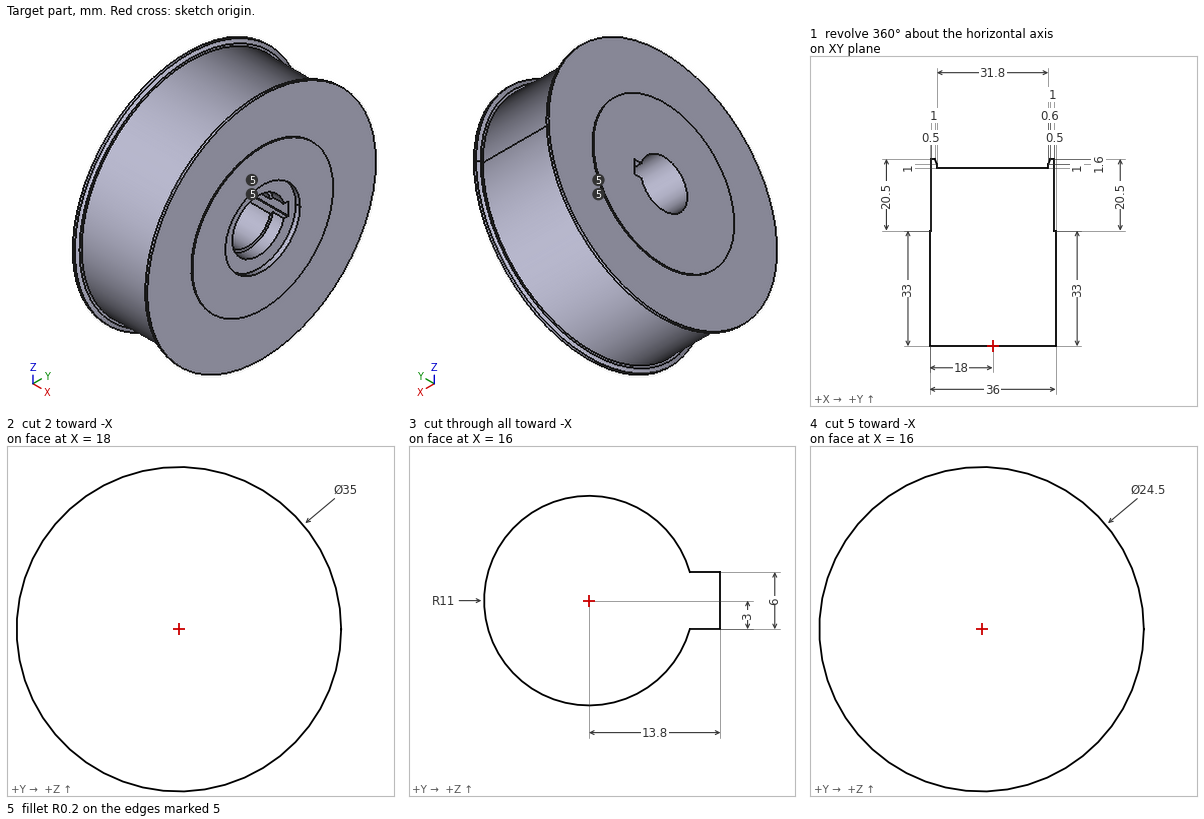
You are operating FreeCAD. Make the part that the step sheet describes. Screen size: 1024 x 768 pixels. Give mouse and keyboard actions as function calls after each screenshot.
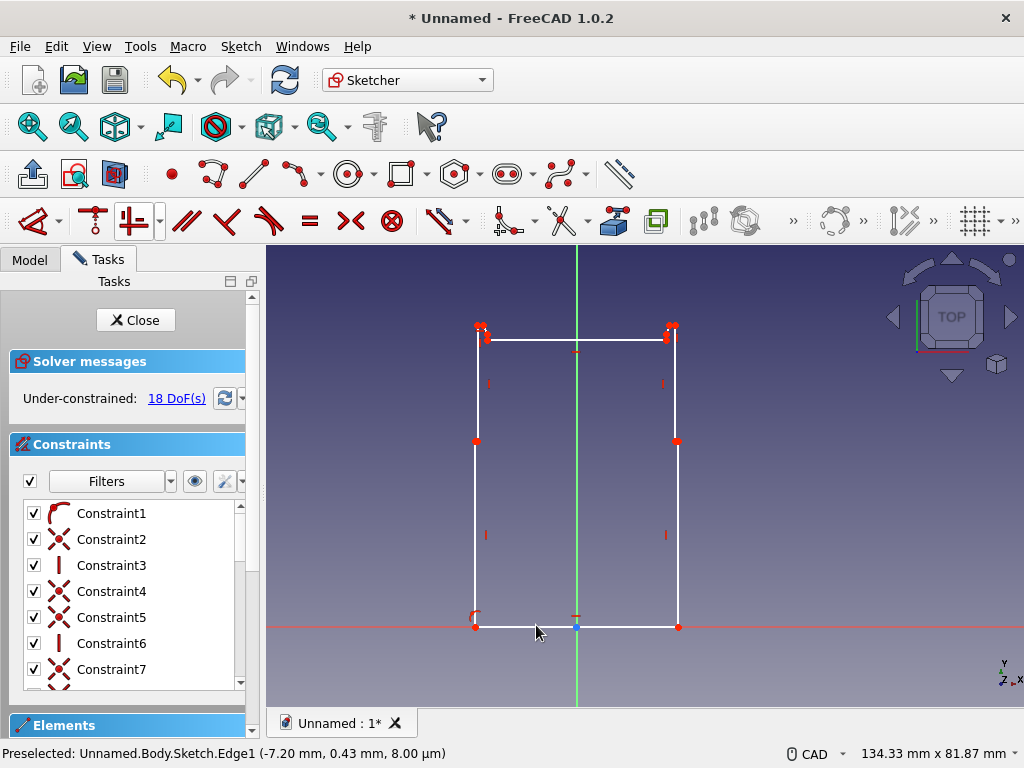
scroll(677, 442, up, 12)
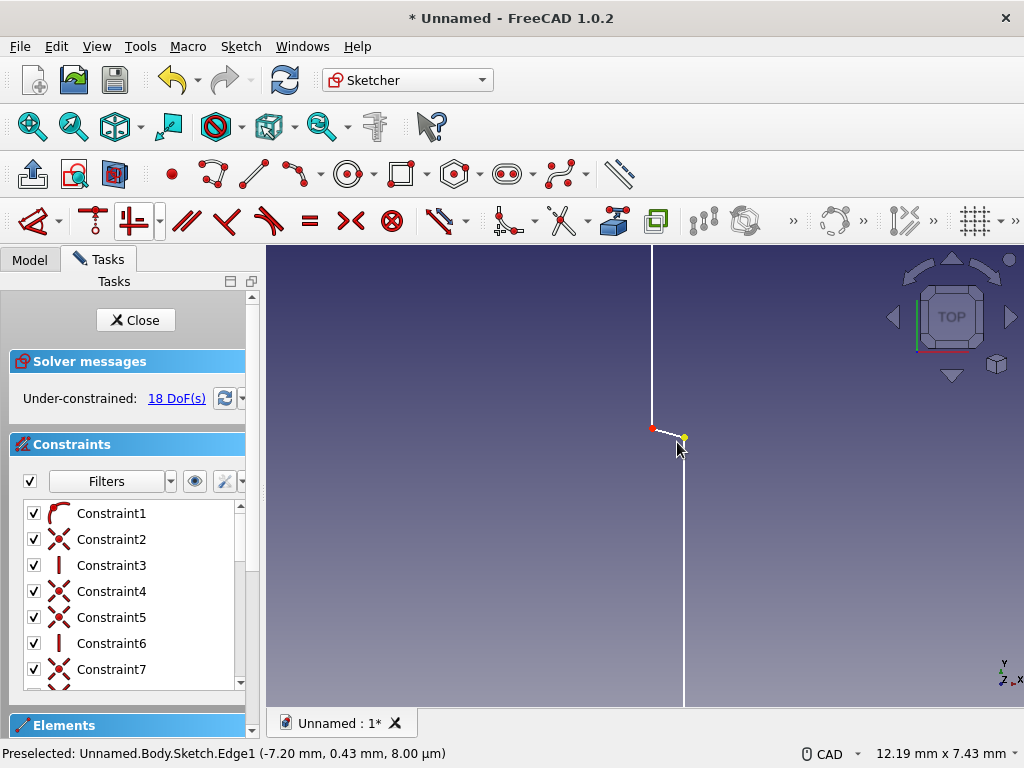
click(668, 433)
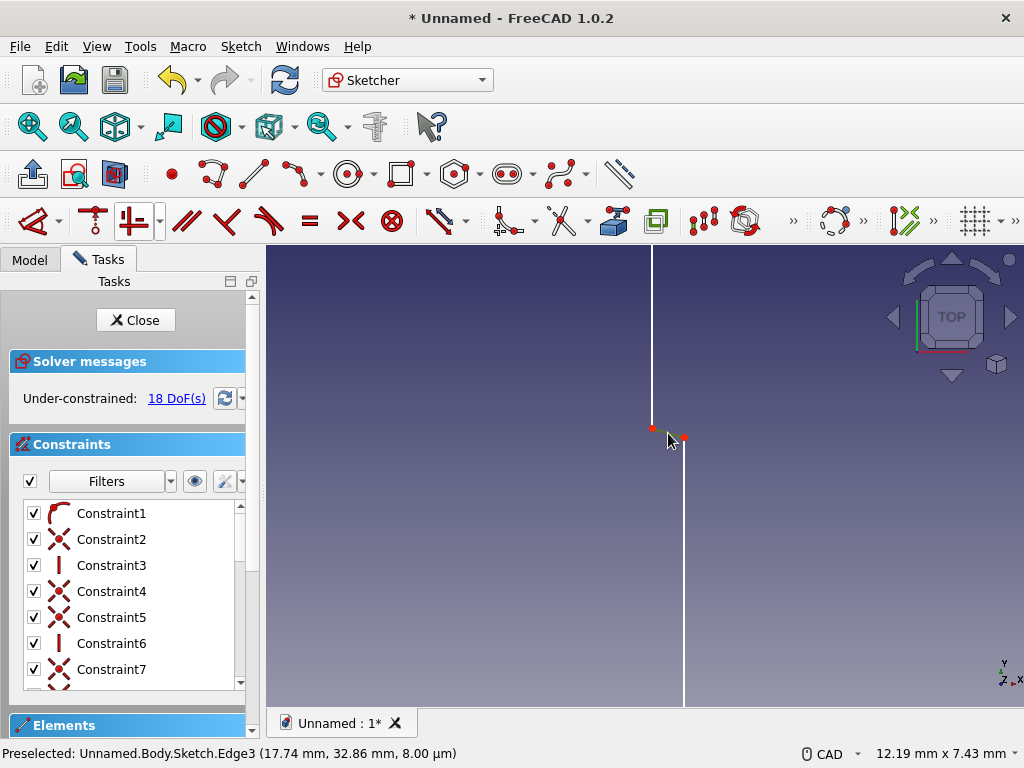
key(h)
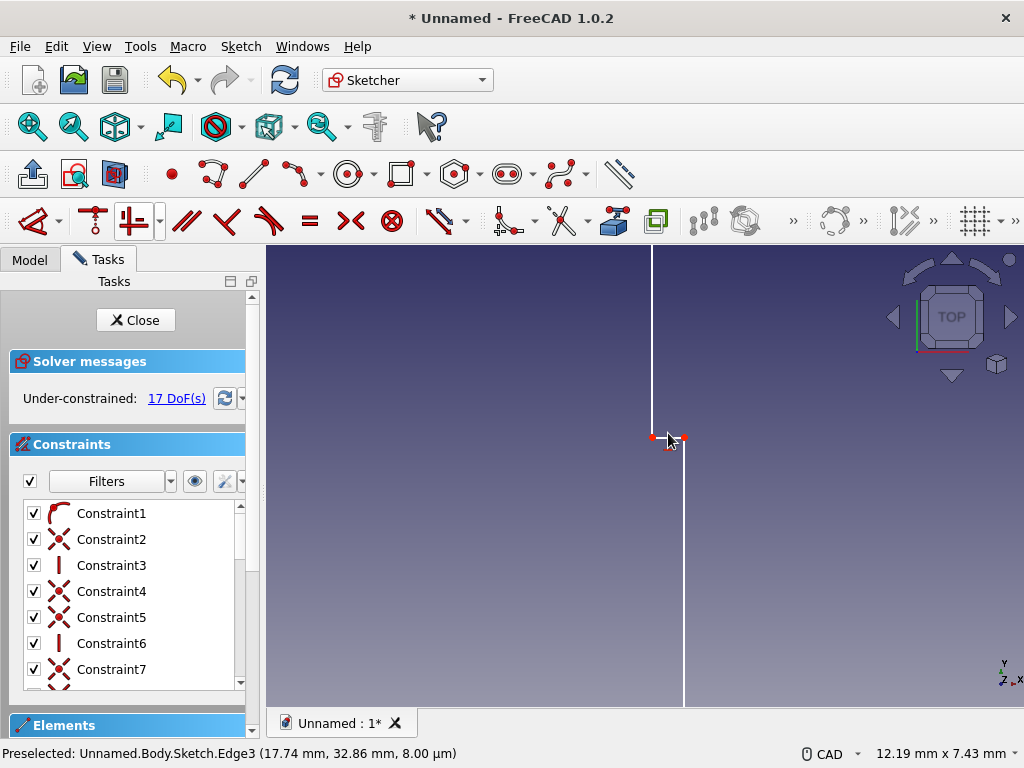
scroll(677, 442, down, 12)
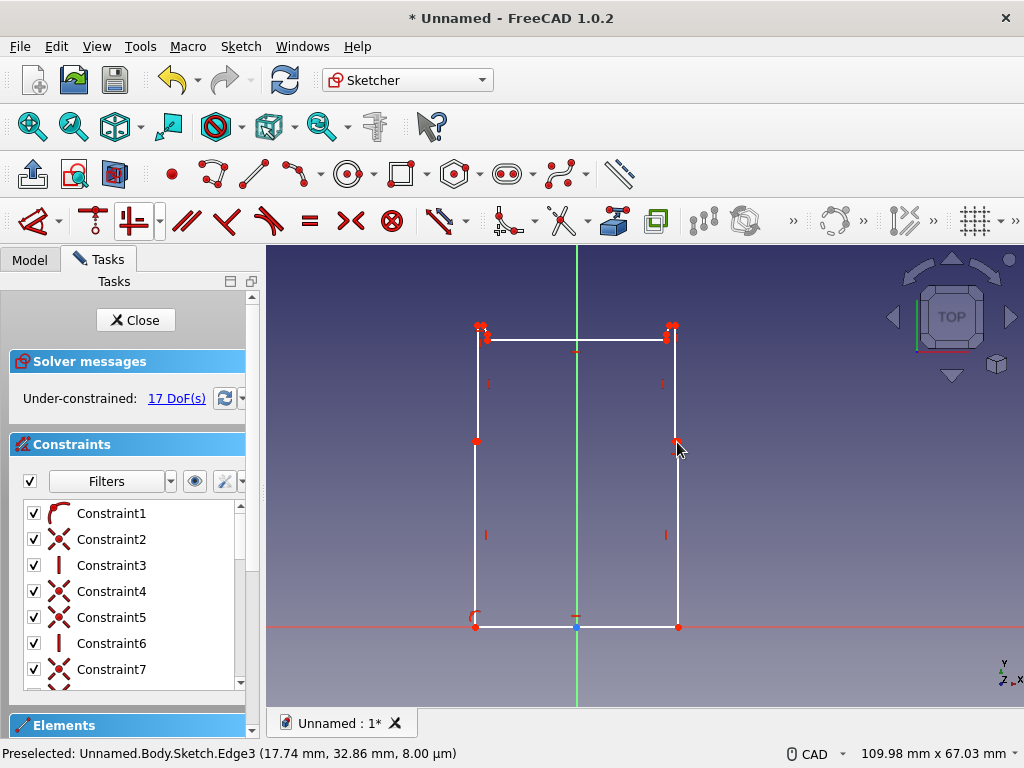
scroll(674, 326, up, 11)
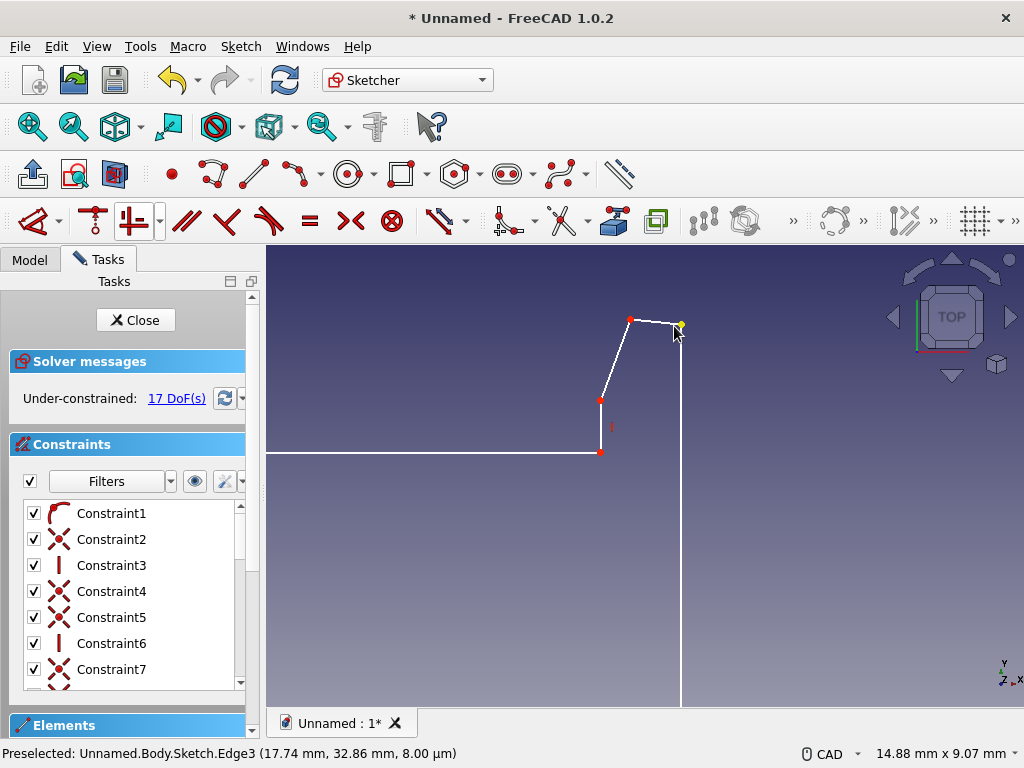
click(666, 323)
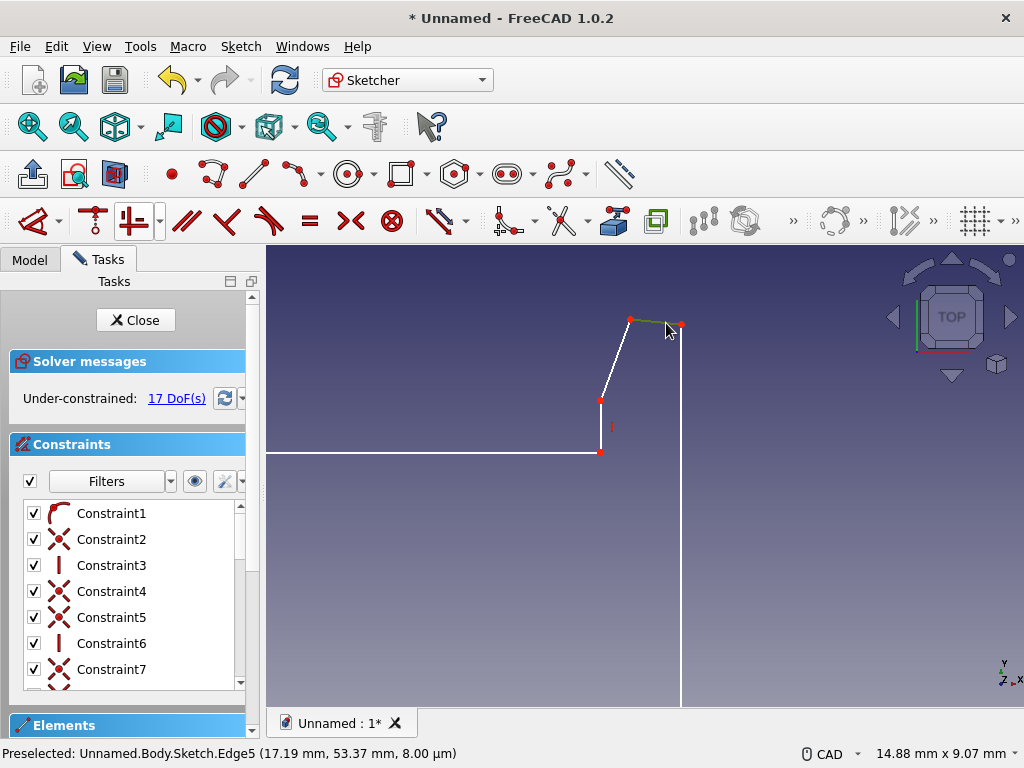
key(h)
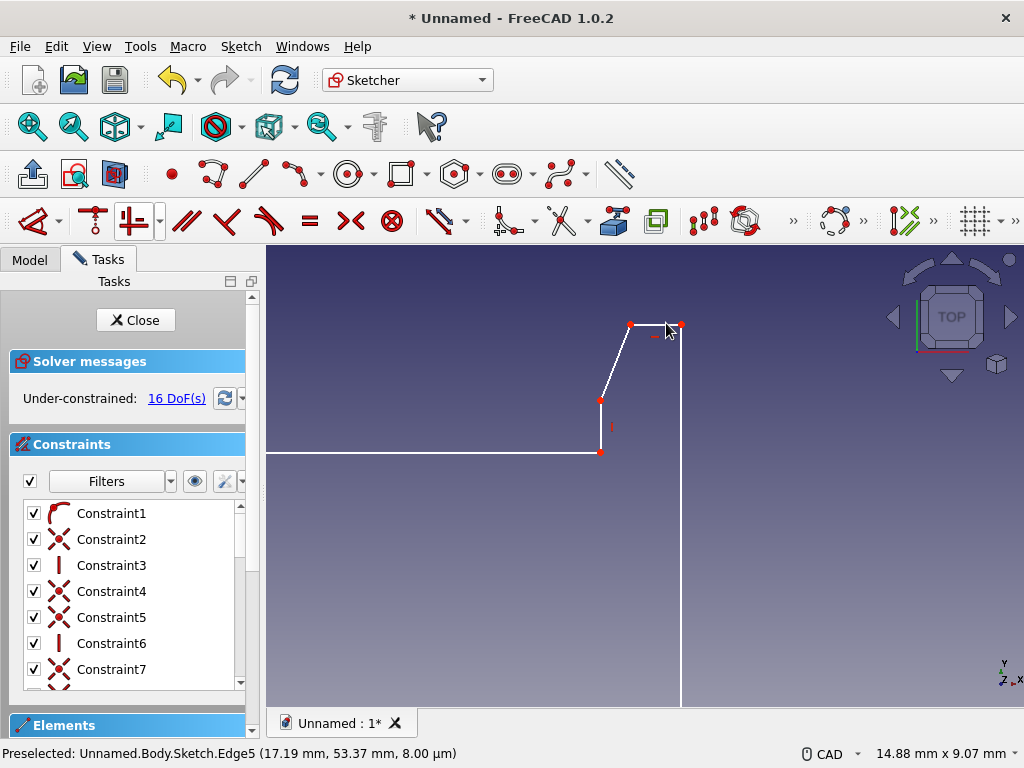
scroll(674, 326, down, 11)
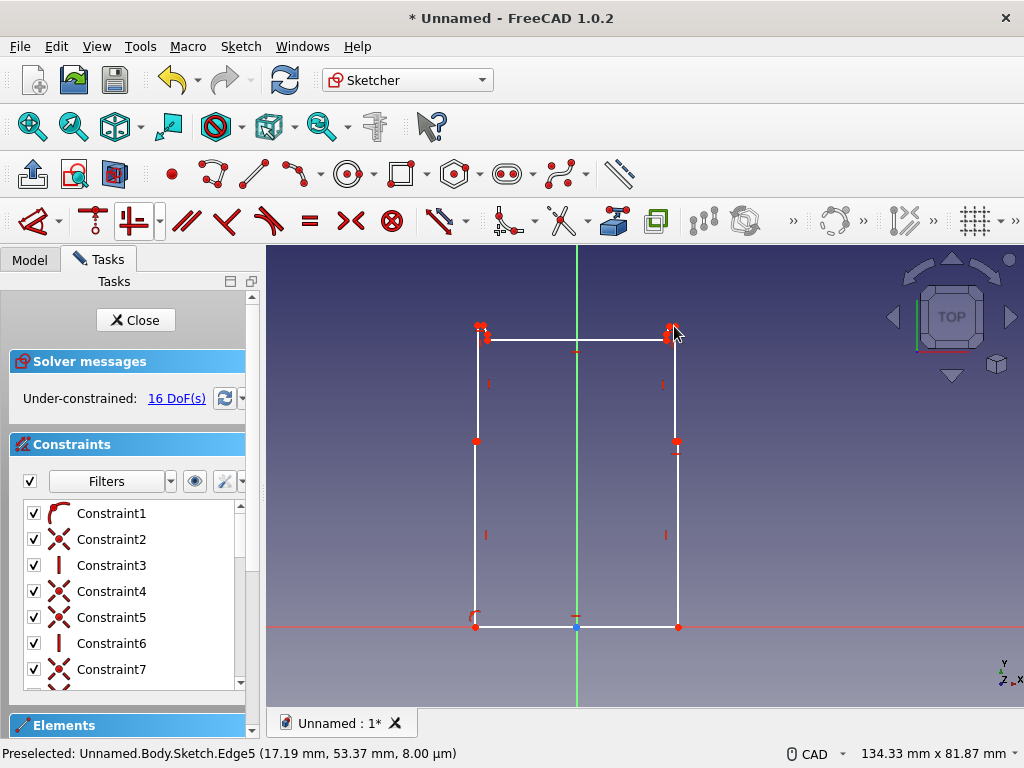
scroll(477, 442, up, 13)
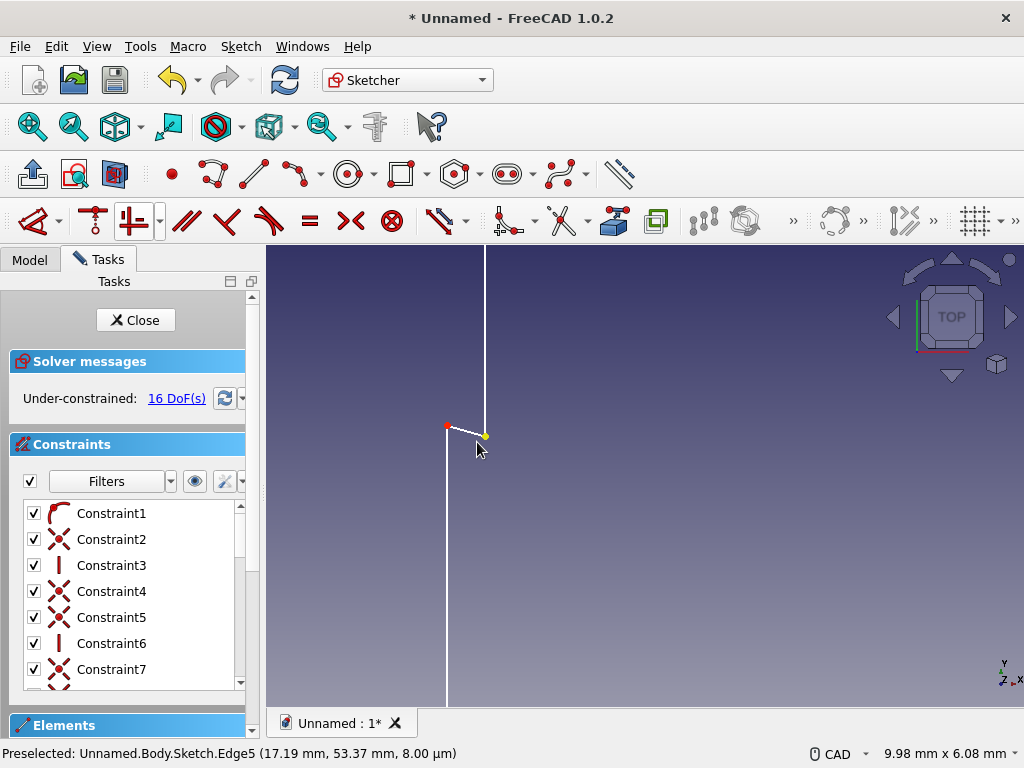
click(470, 432)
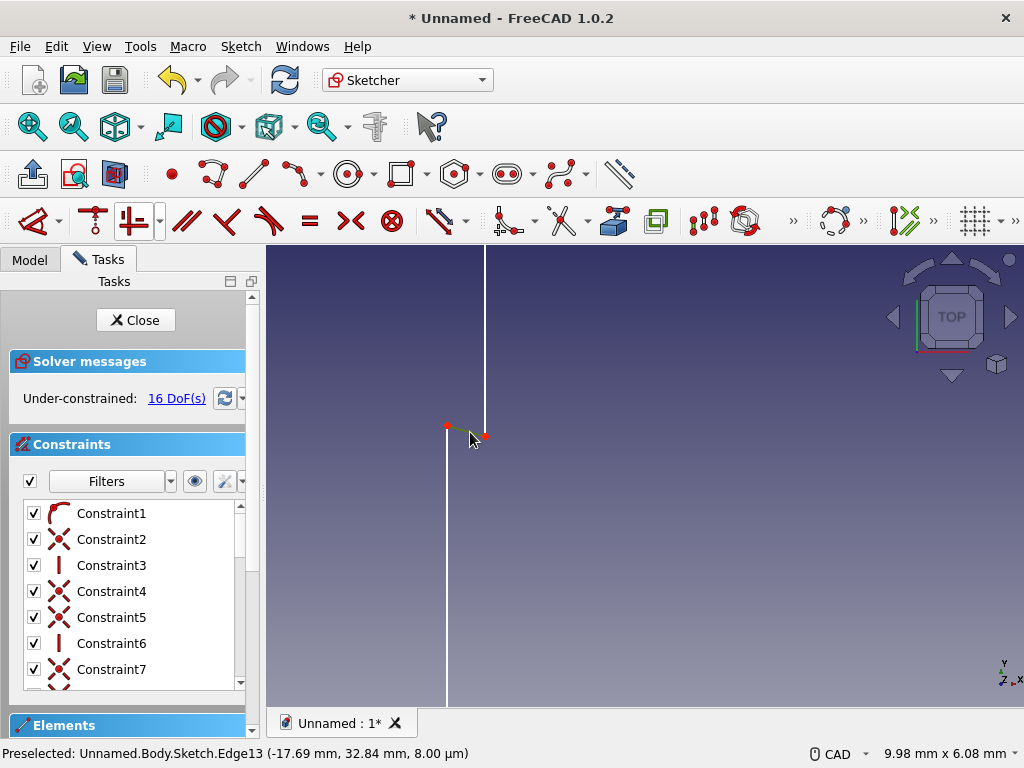
key(h)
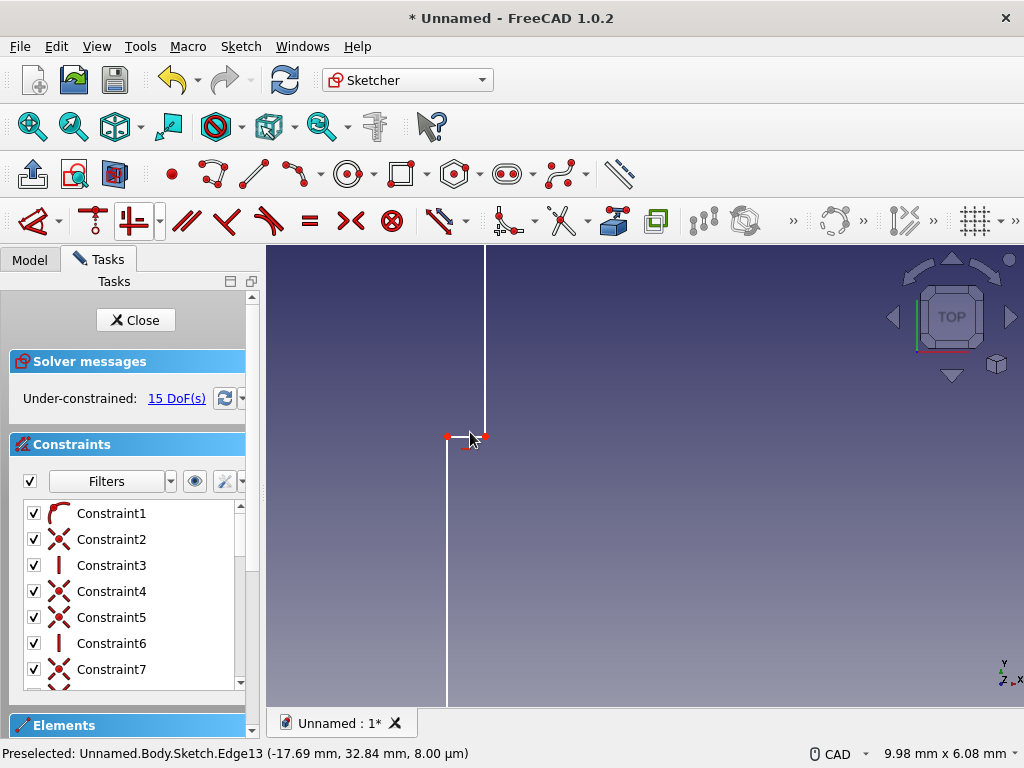
key(d)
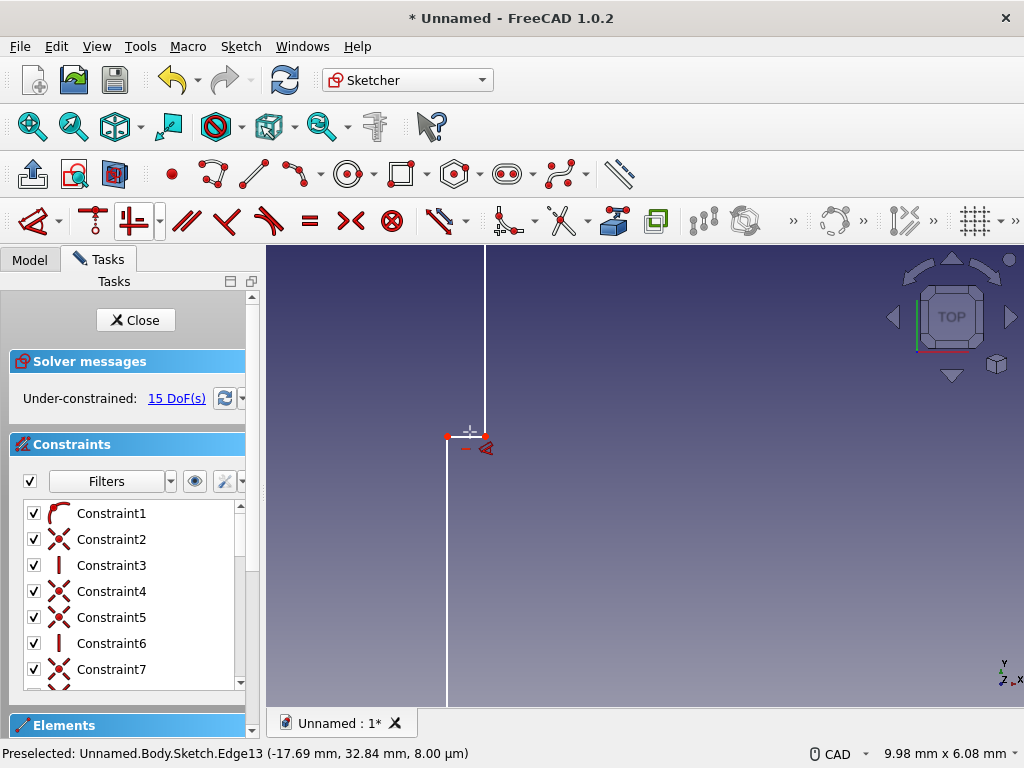
scroll(477, 442, down, 13)